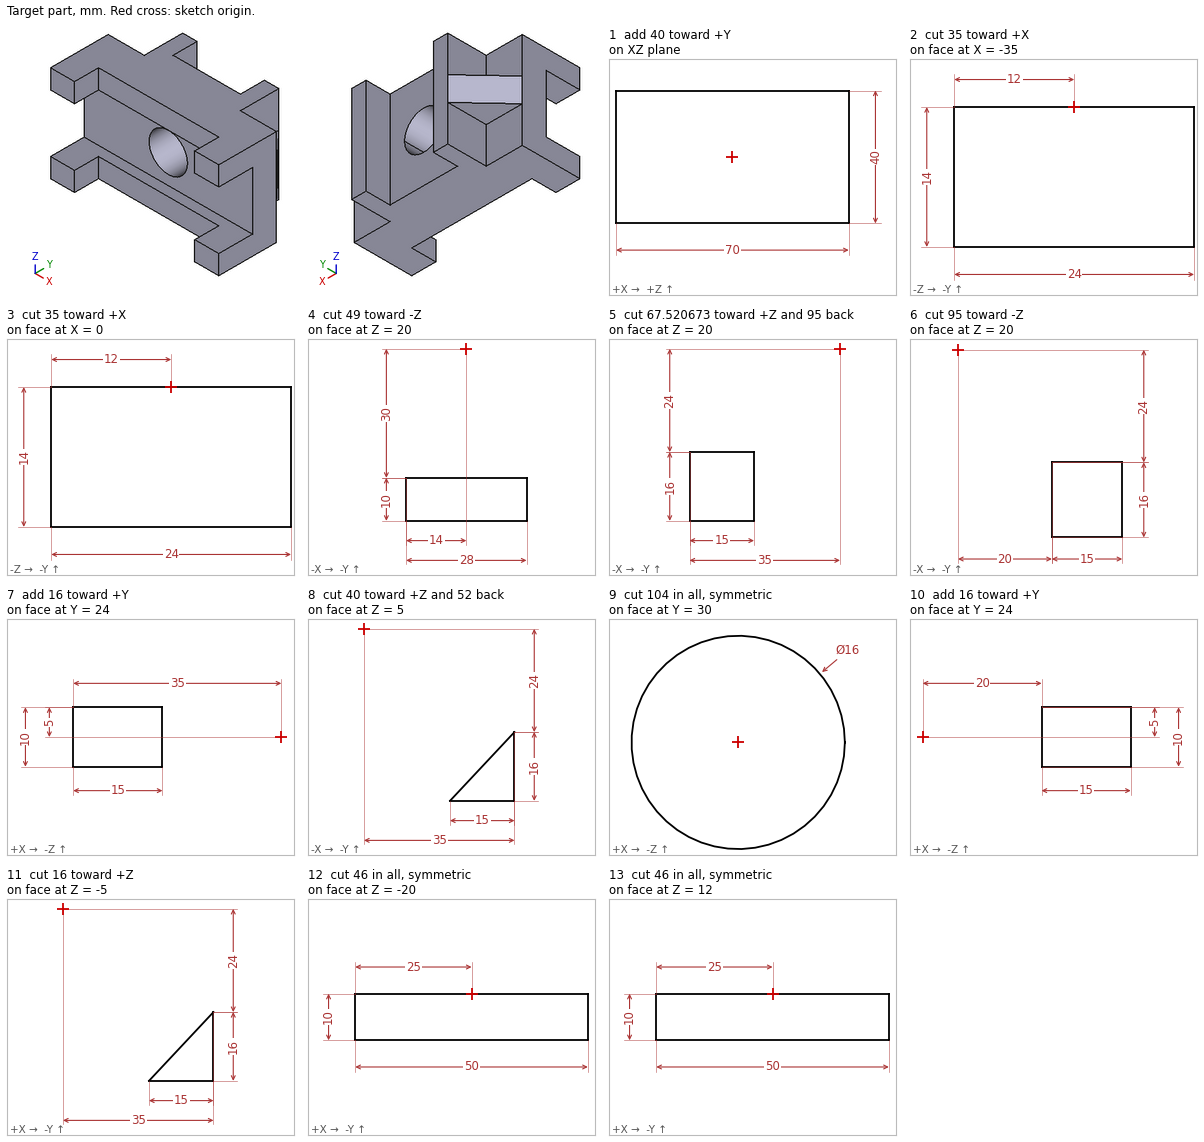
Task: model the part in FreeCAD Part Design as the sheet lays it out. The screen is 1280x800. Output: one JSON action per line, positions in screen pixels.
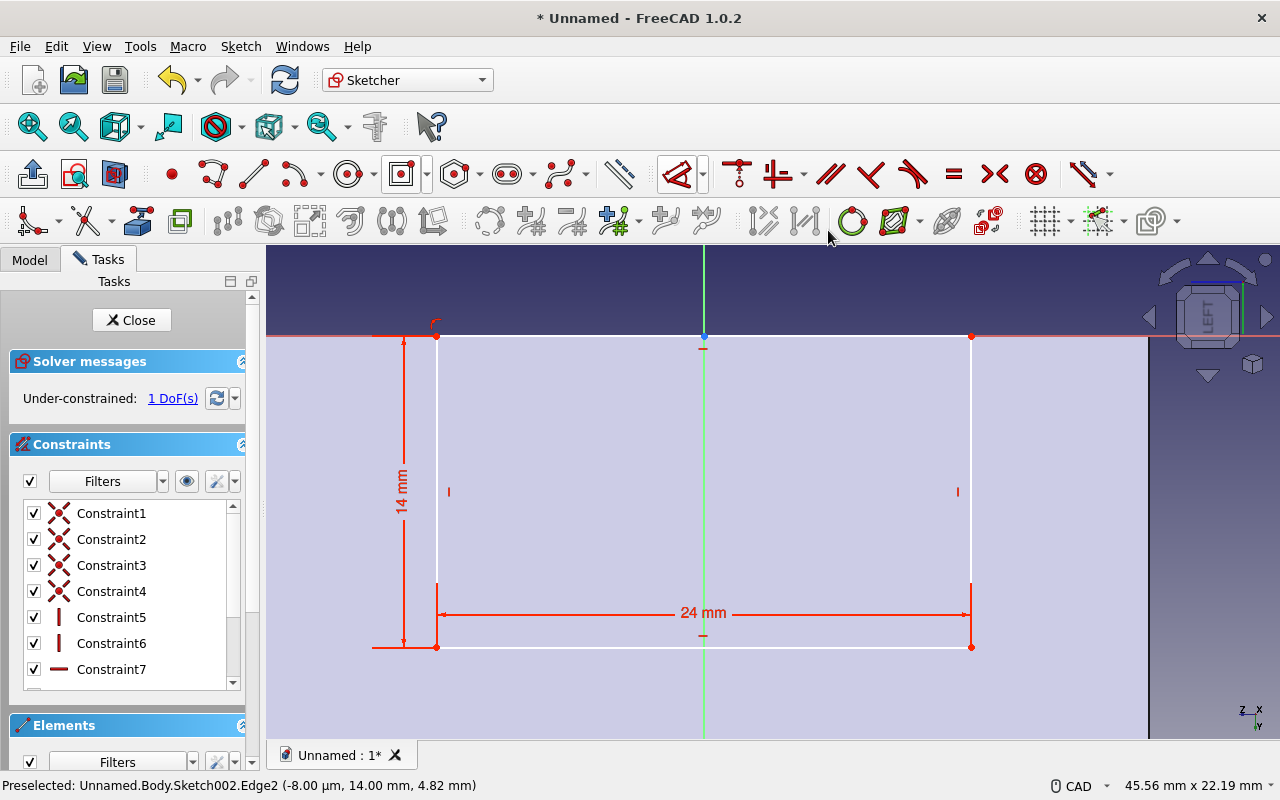
{"action": "left_click", "coordinate": [437, 336]}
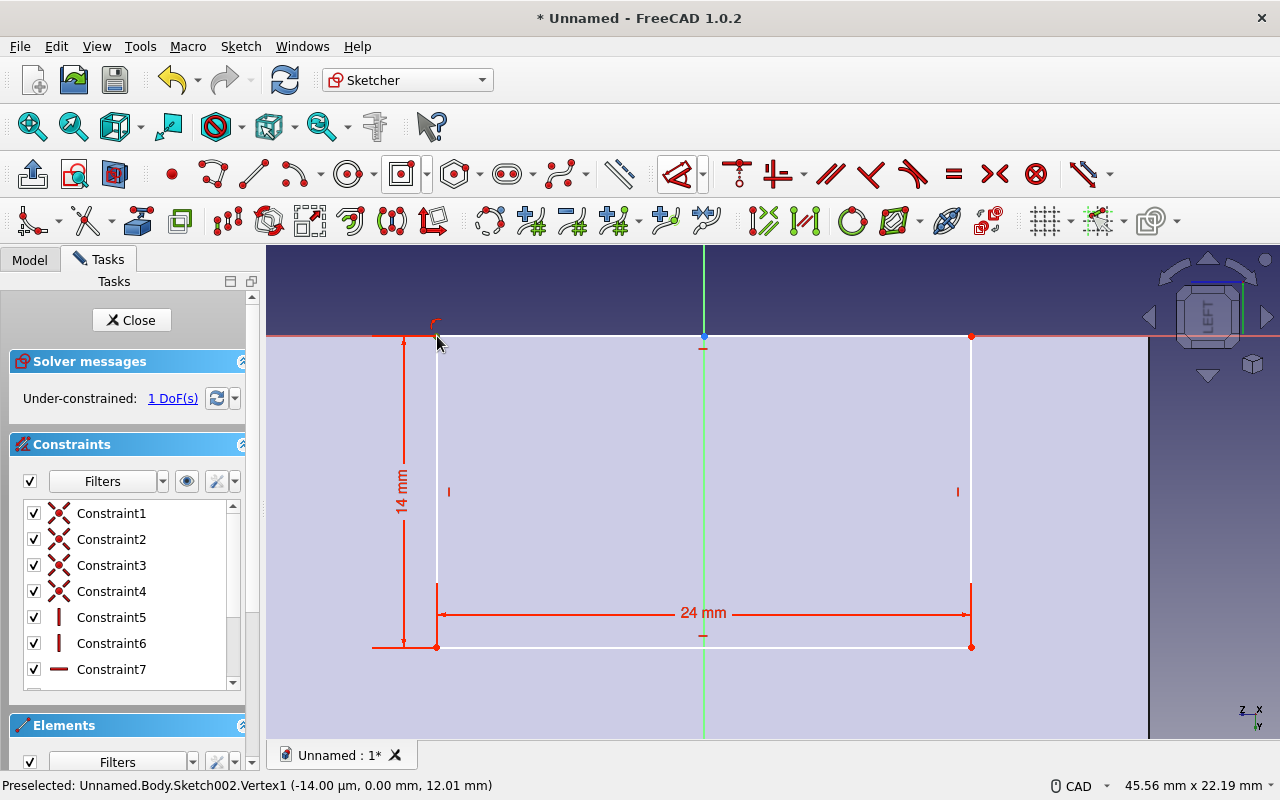
{"action": "key", "text": "l"}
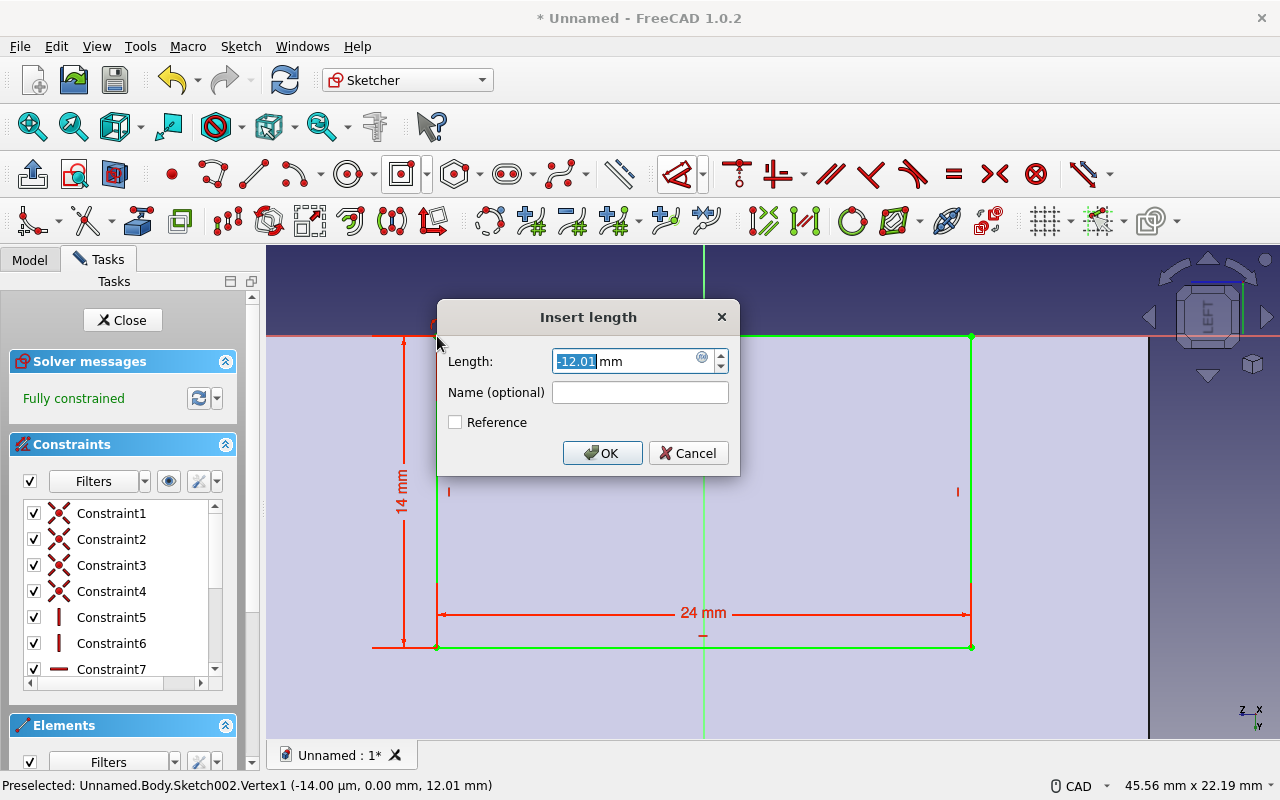
{"action": "type", "text": "-12"}
{"action": "key", "text": "Return"}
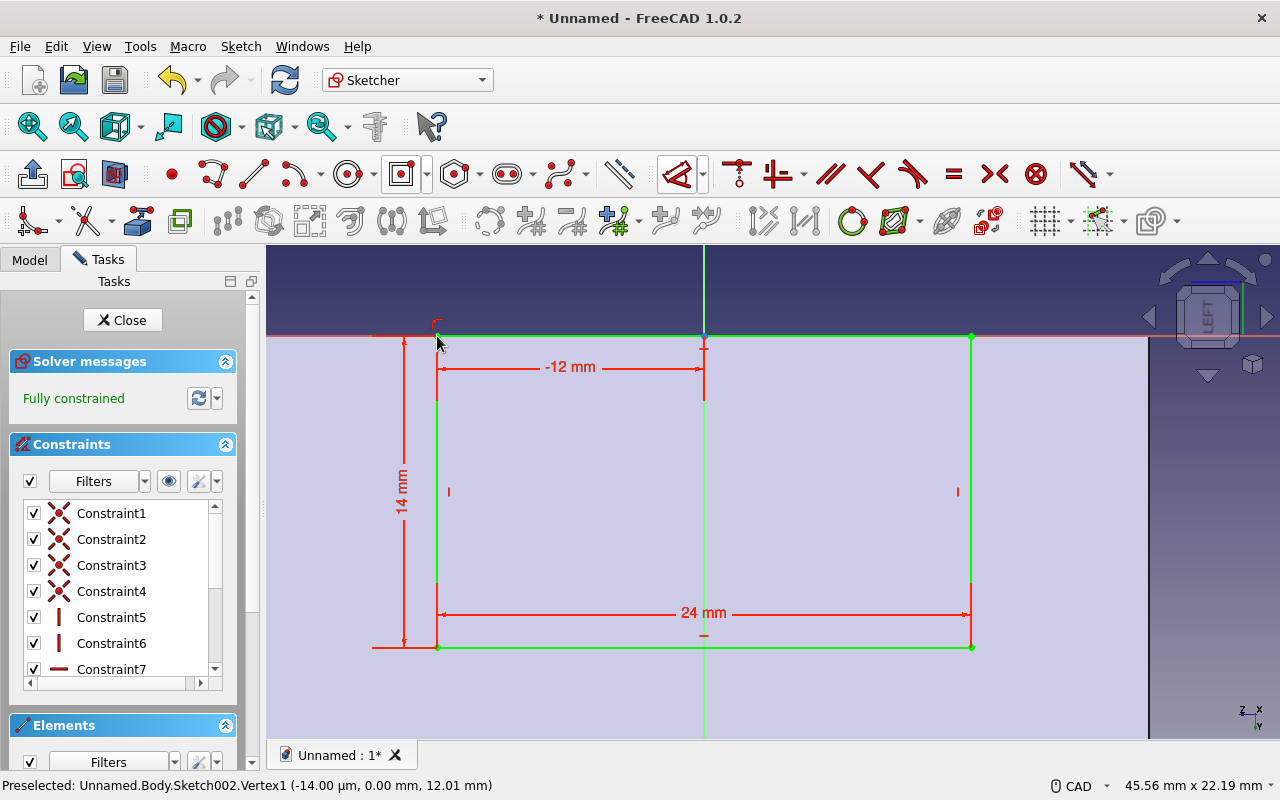
{"action": "left_click", "coordinate": [123, 320]}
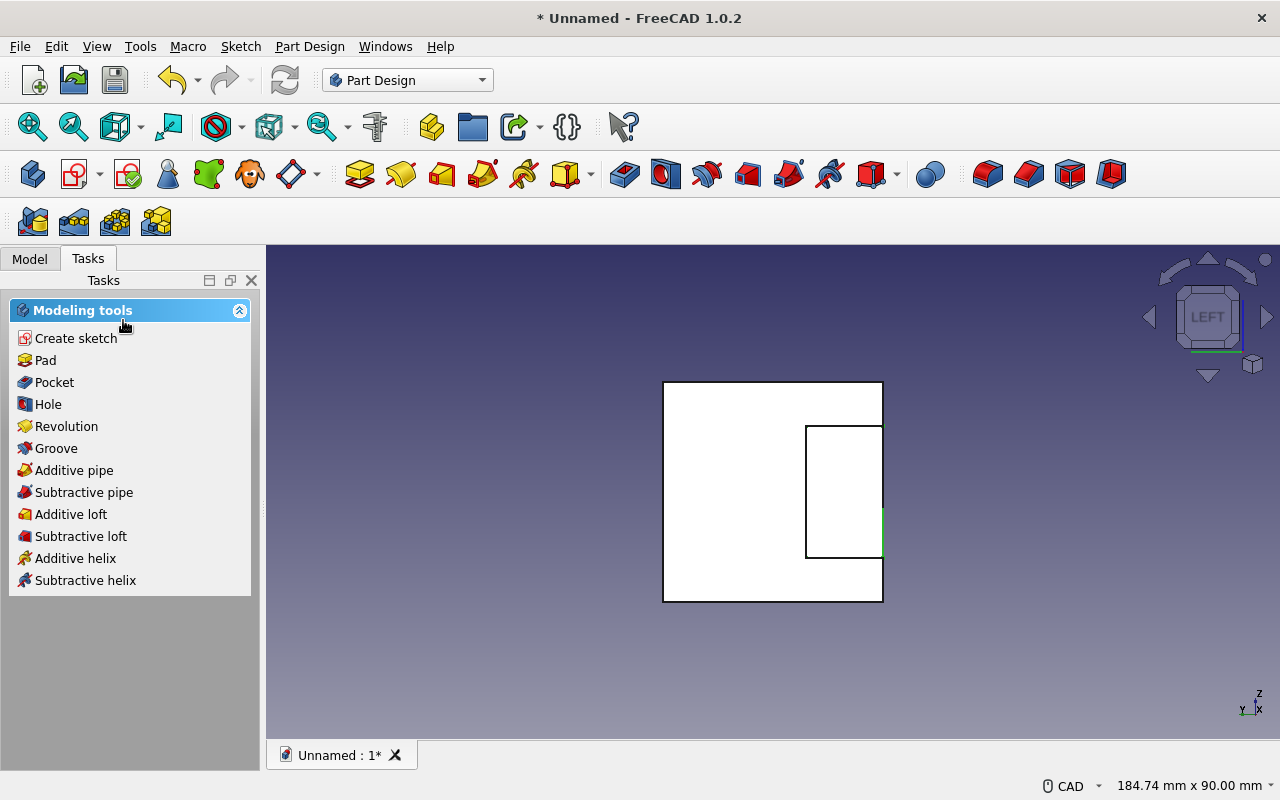
{"action": "left_click", "coordinate": [625, 174]}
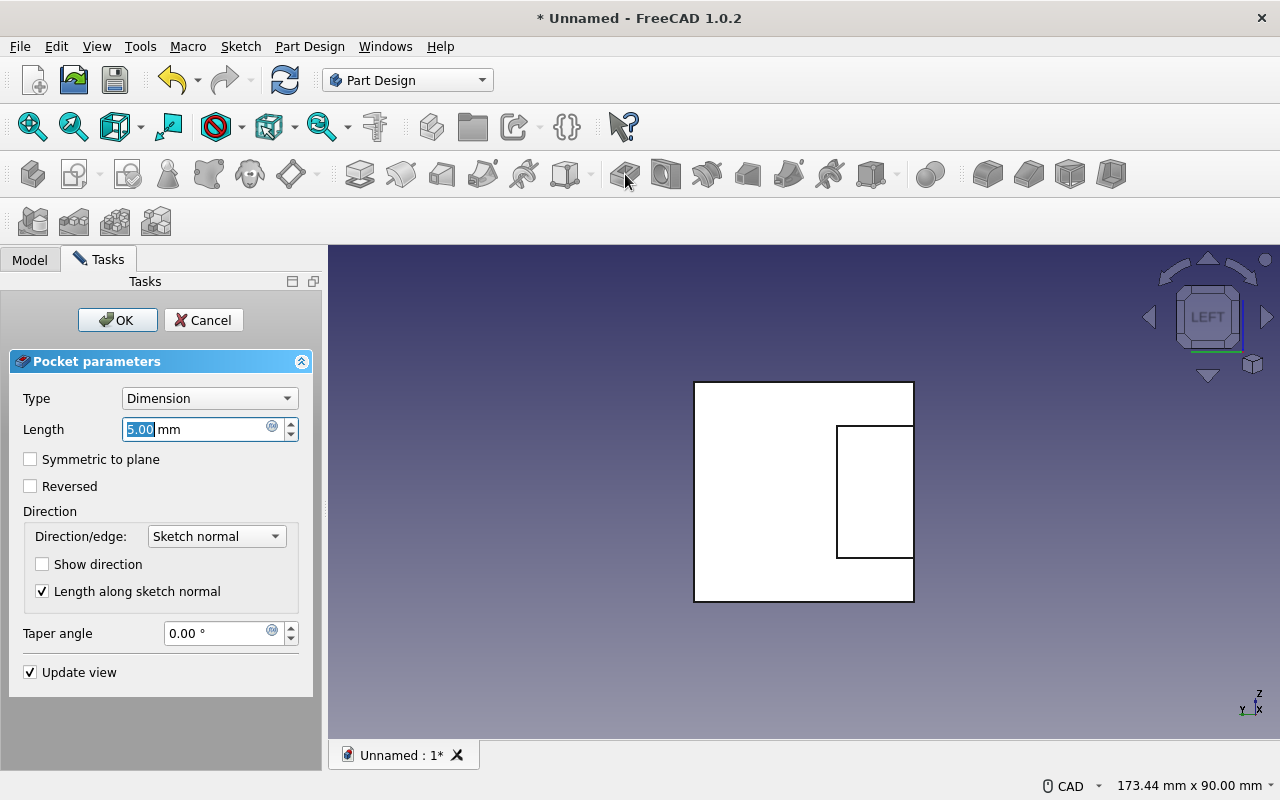
{"action": "type", "text": "35"}
{"action": "key", "text": "Tab"}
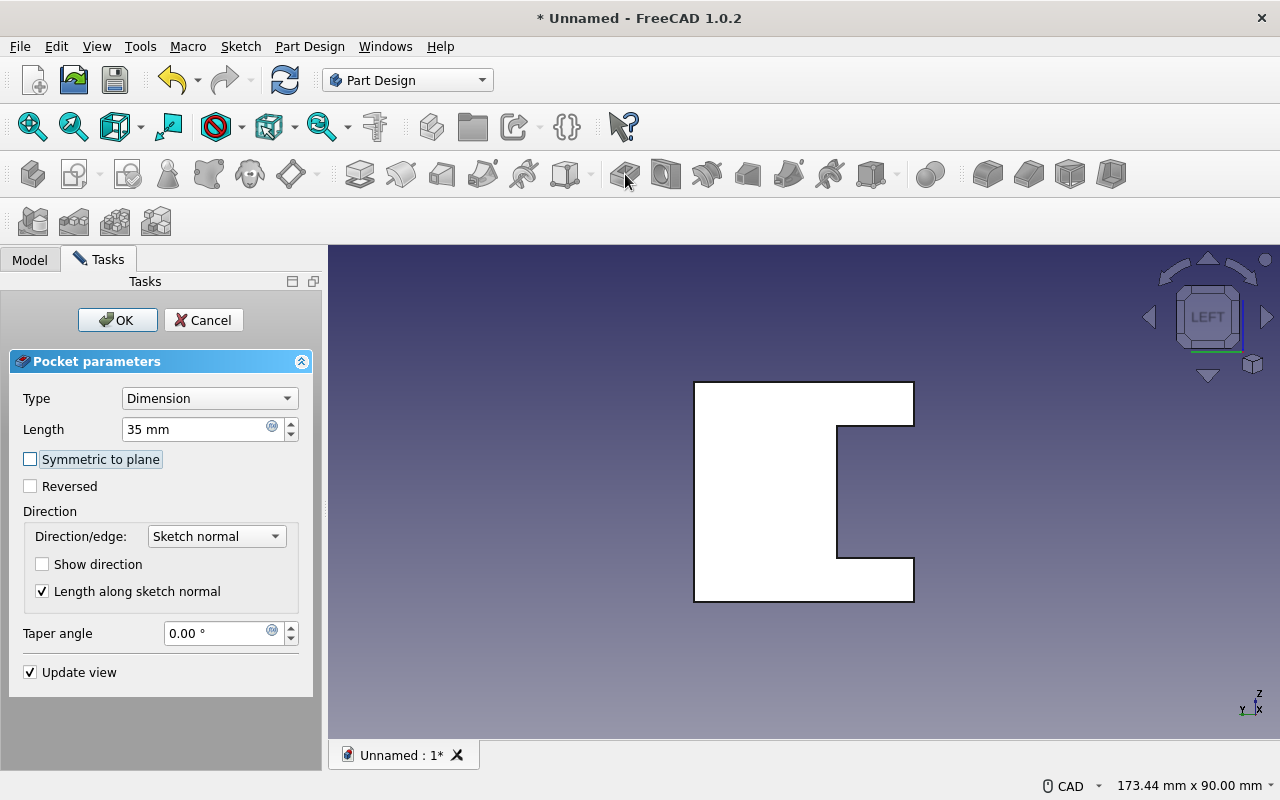
{"action": "left_click", "coordinate": [118, 320]}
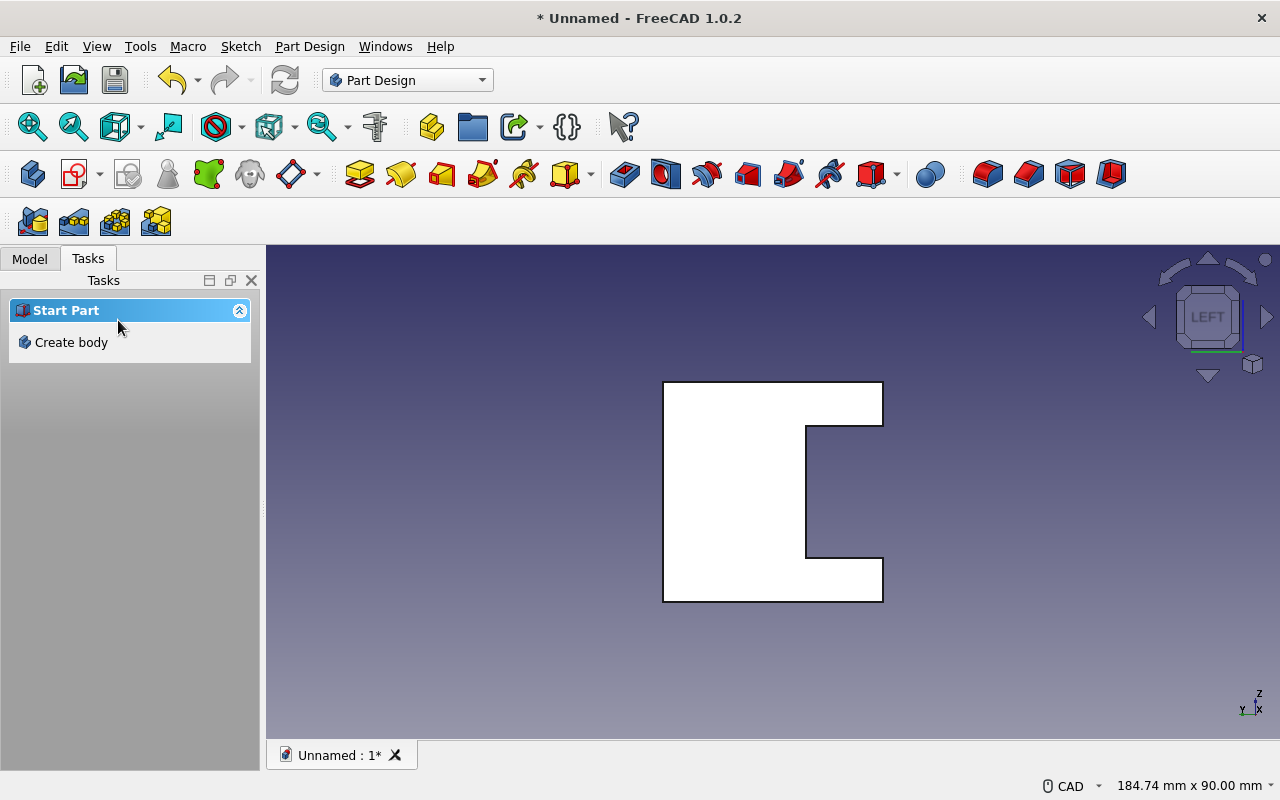
{"action": "key", "text": "v f"}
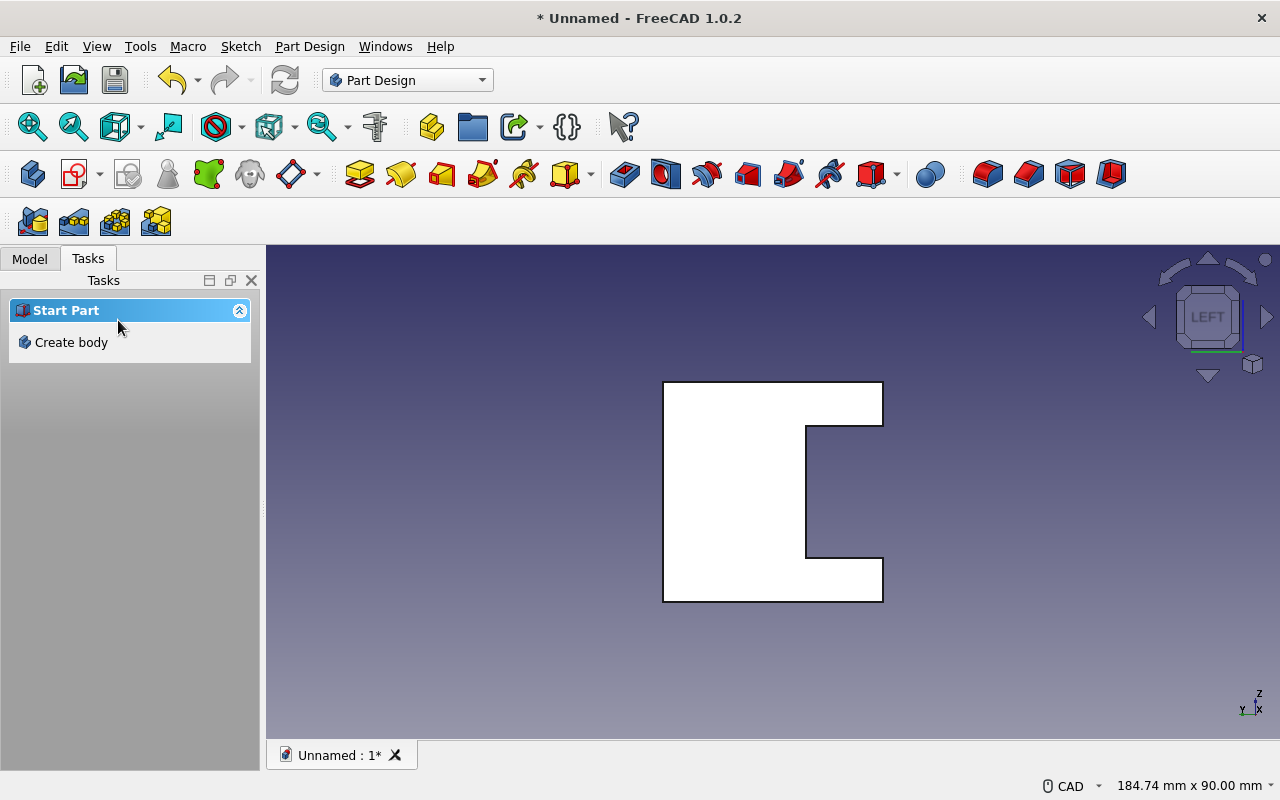
{"action": "key", "text": "0"}